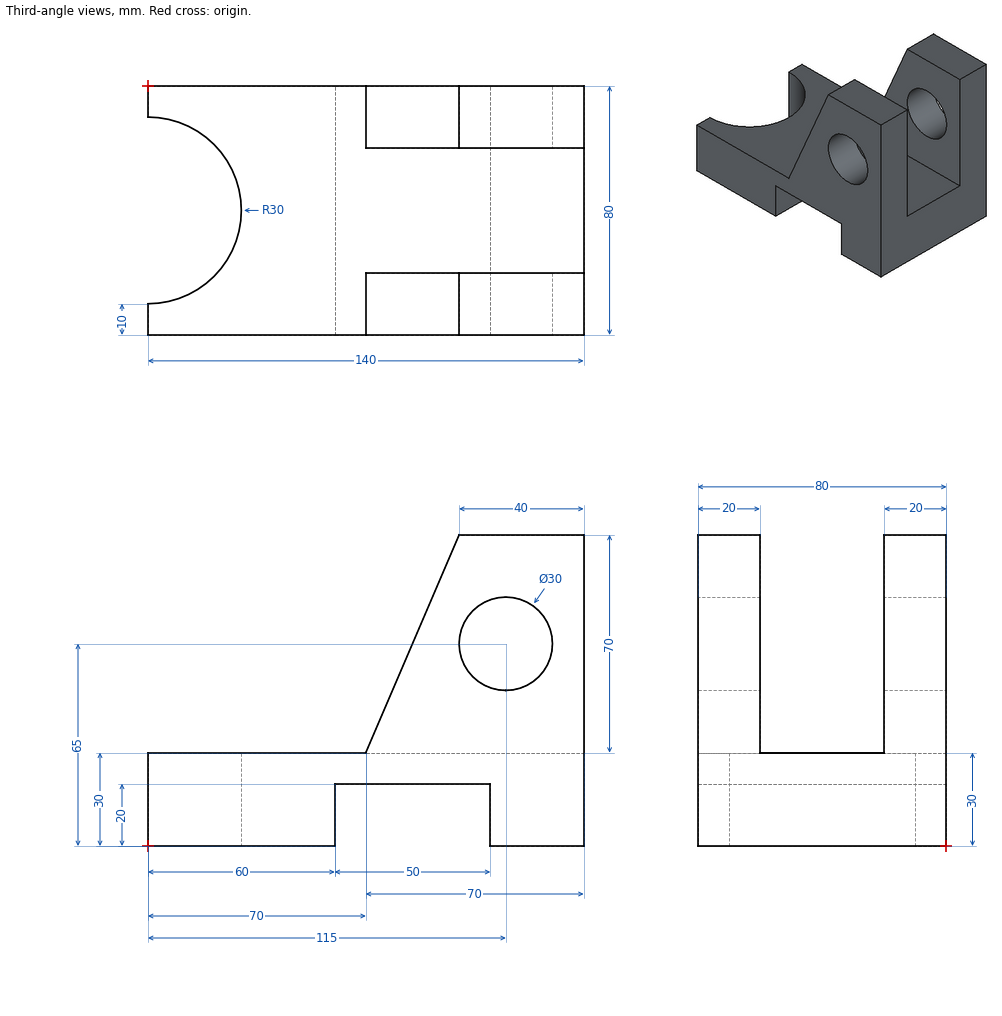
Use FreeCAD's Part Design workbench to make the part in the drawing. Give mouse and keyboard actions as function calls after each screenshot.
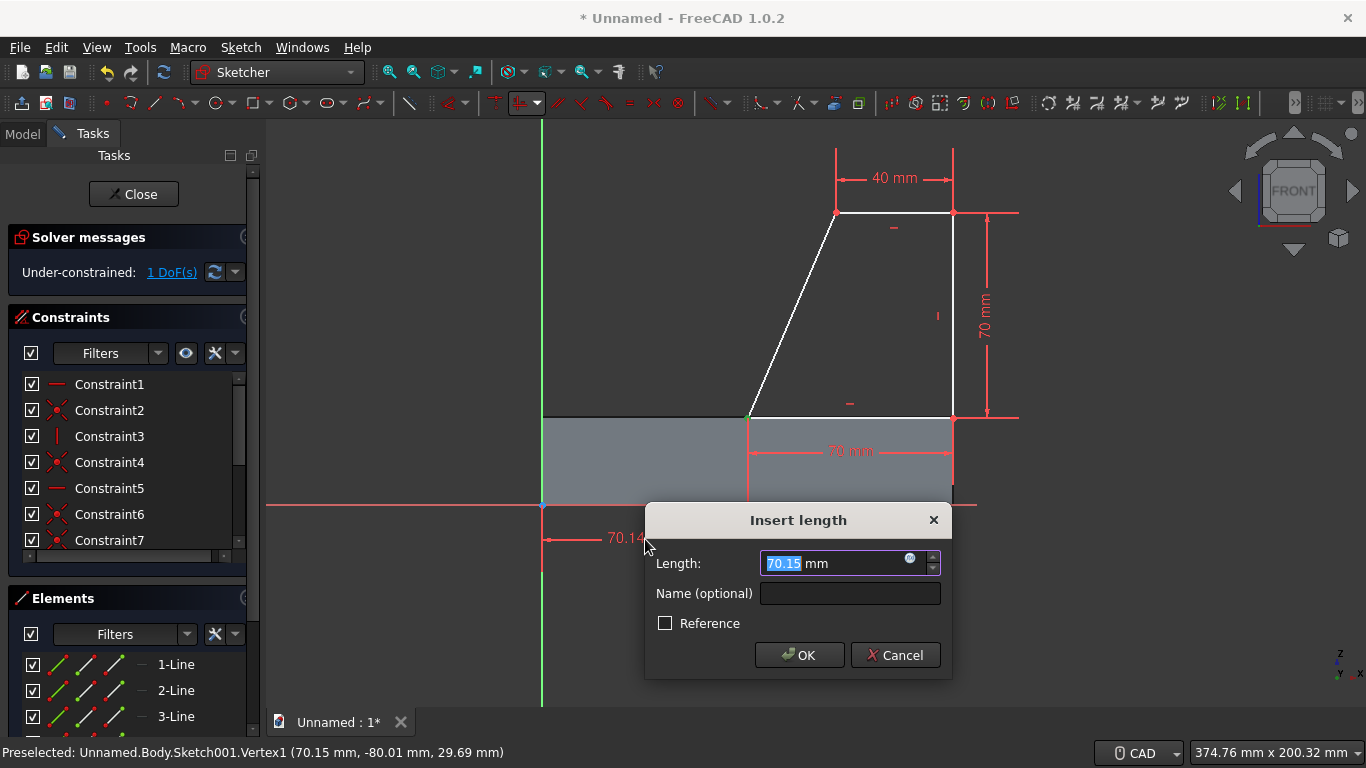
text(70)
key(Return)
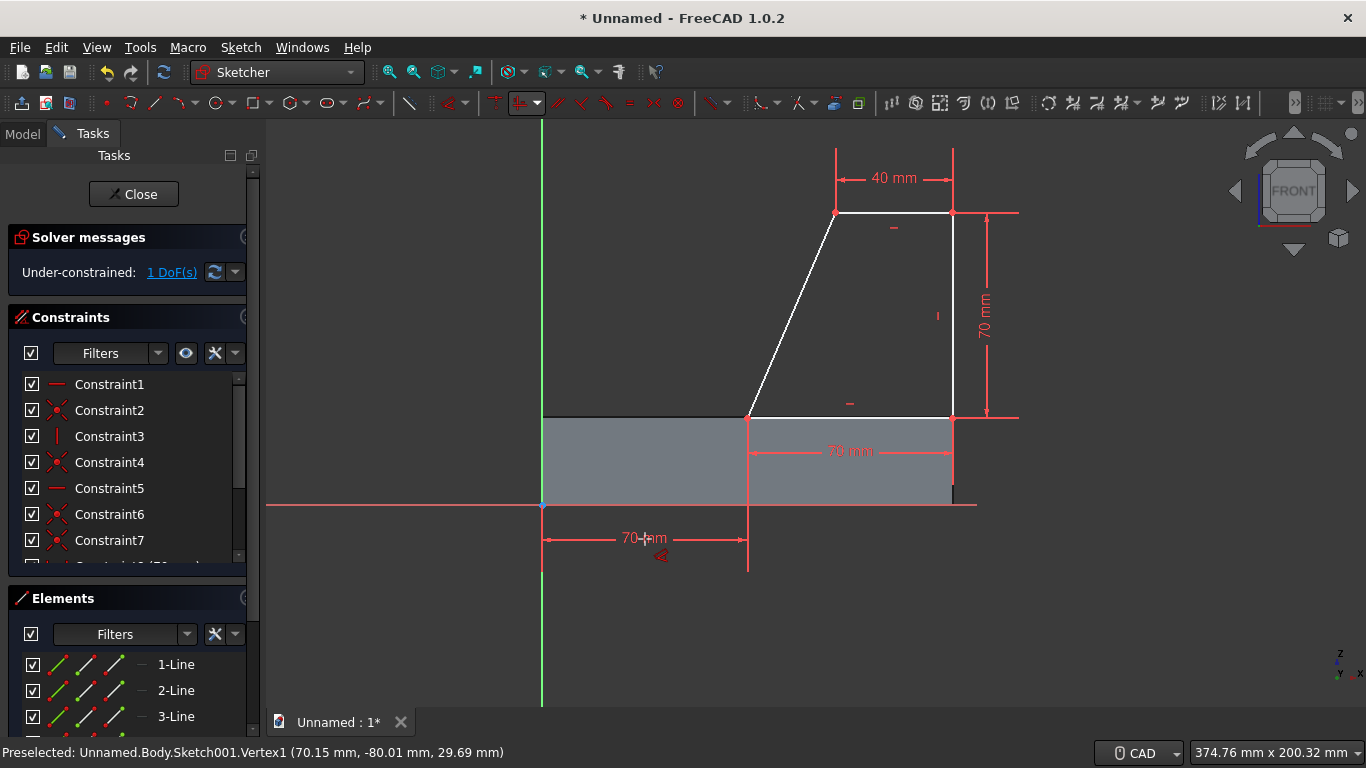
click(748, 418)
click(508, 462)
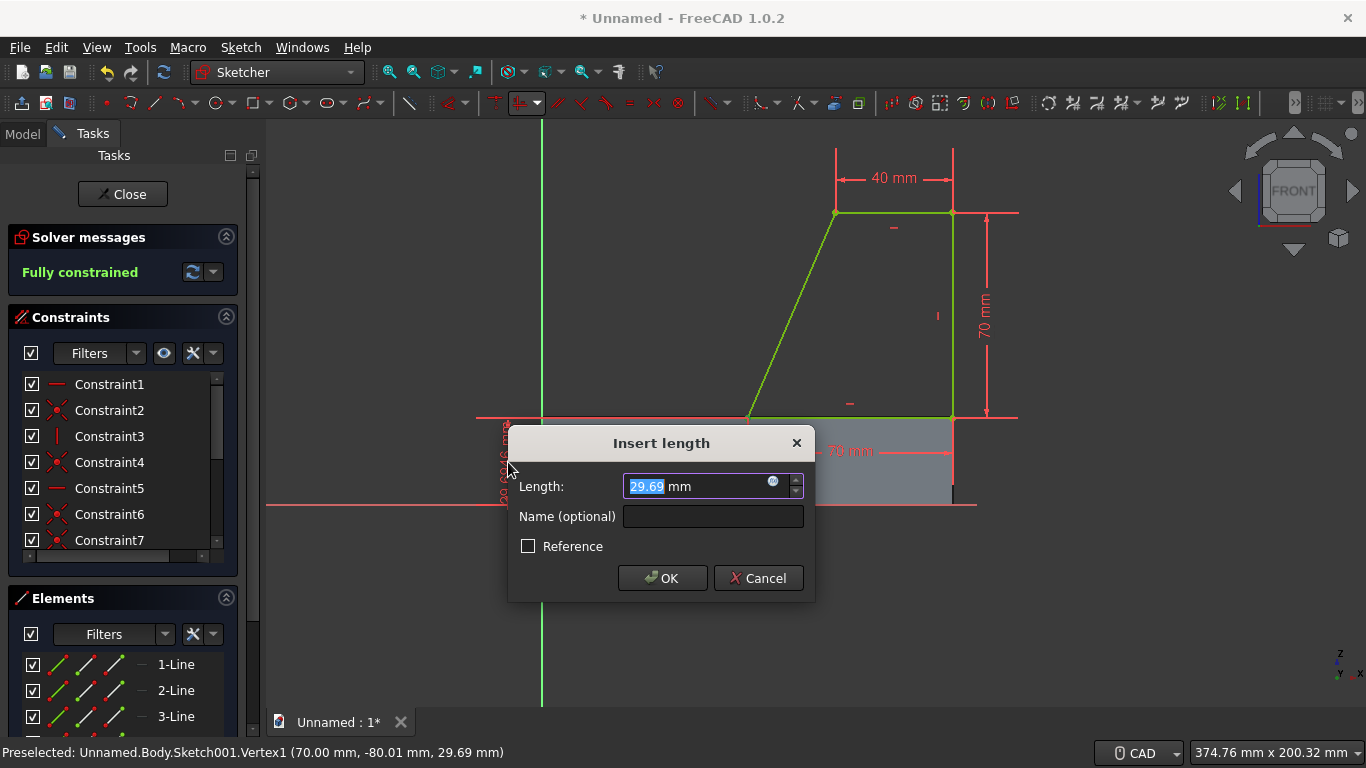
text(30)
key(Return)
key(Escape)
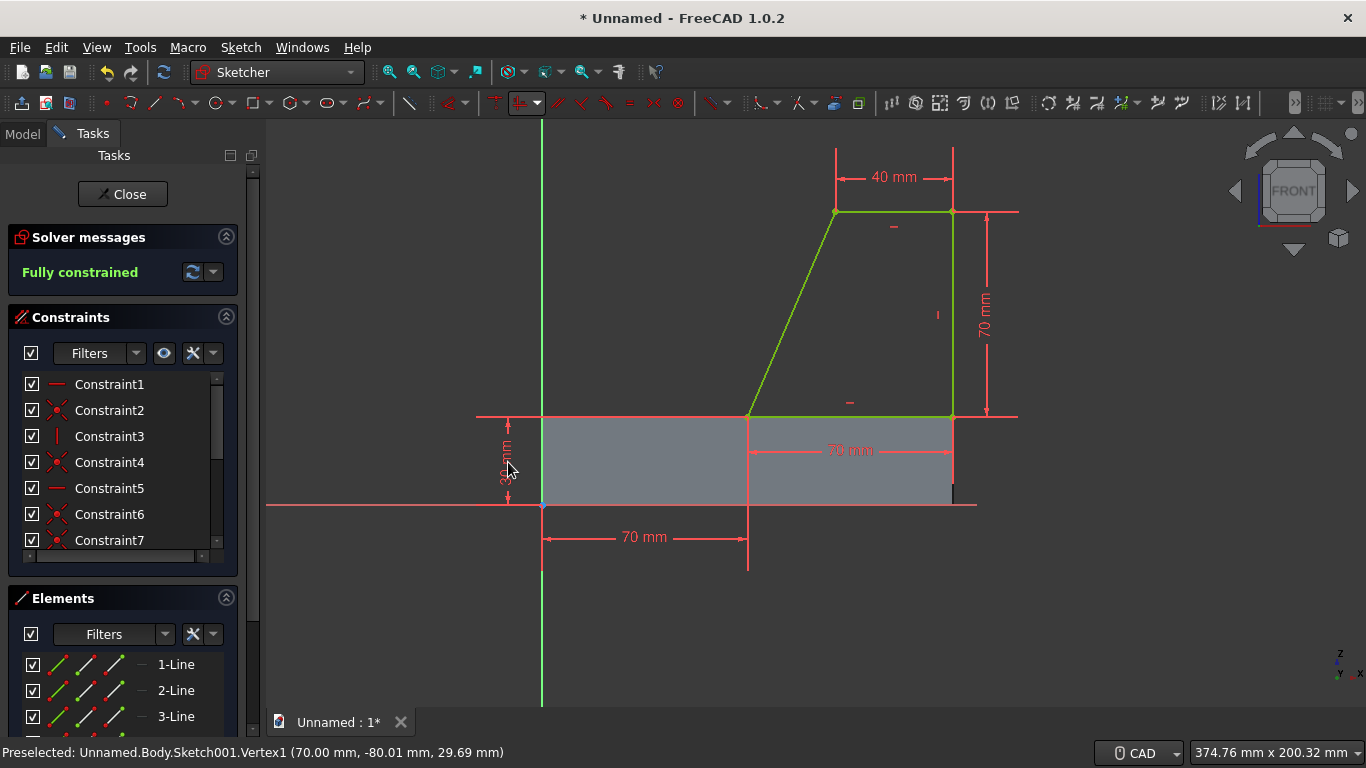
click(123, 194)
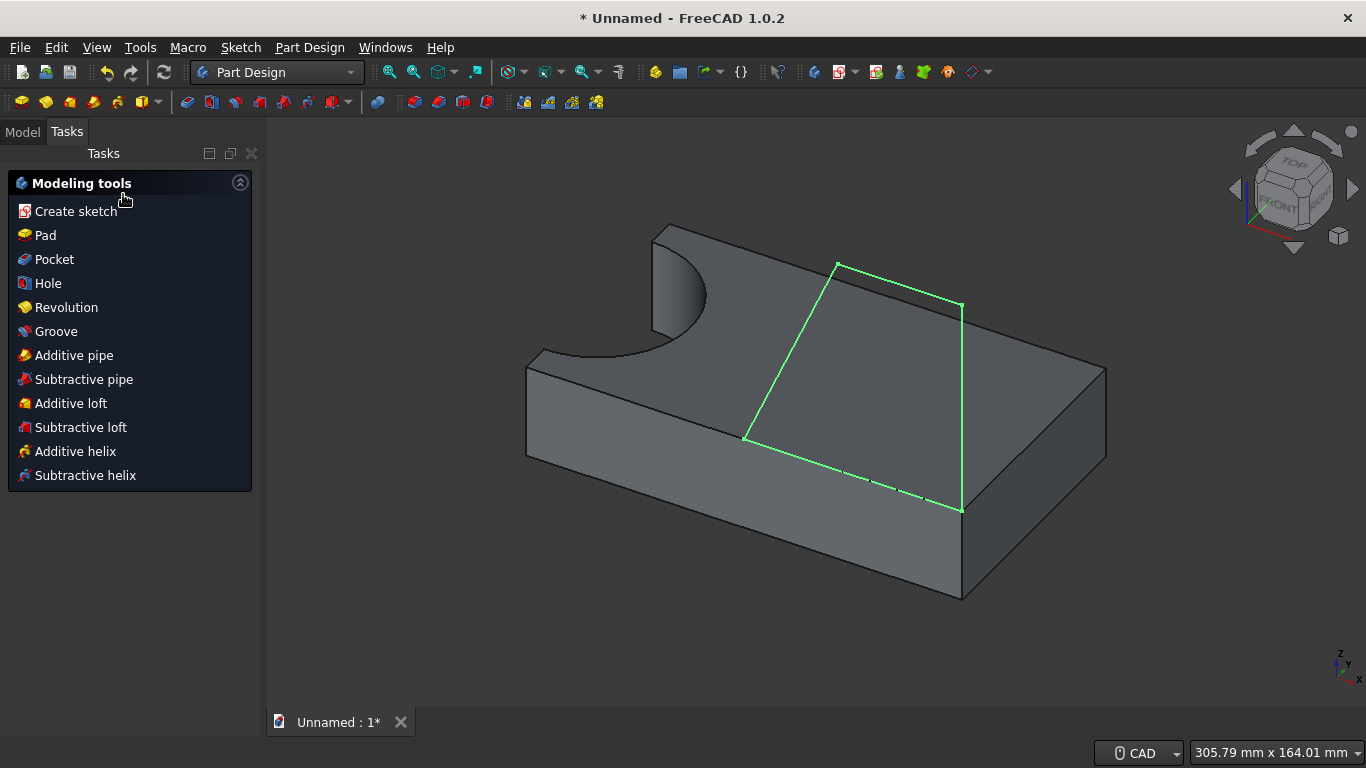
click(22, 102)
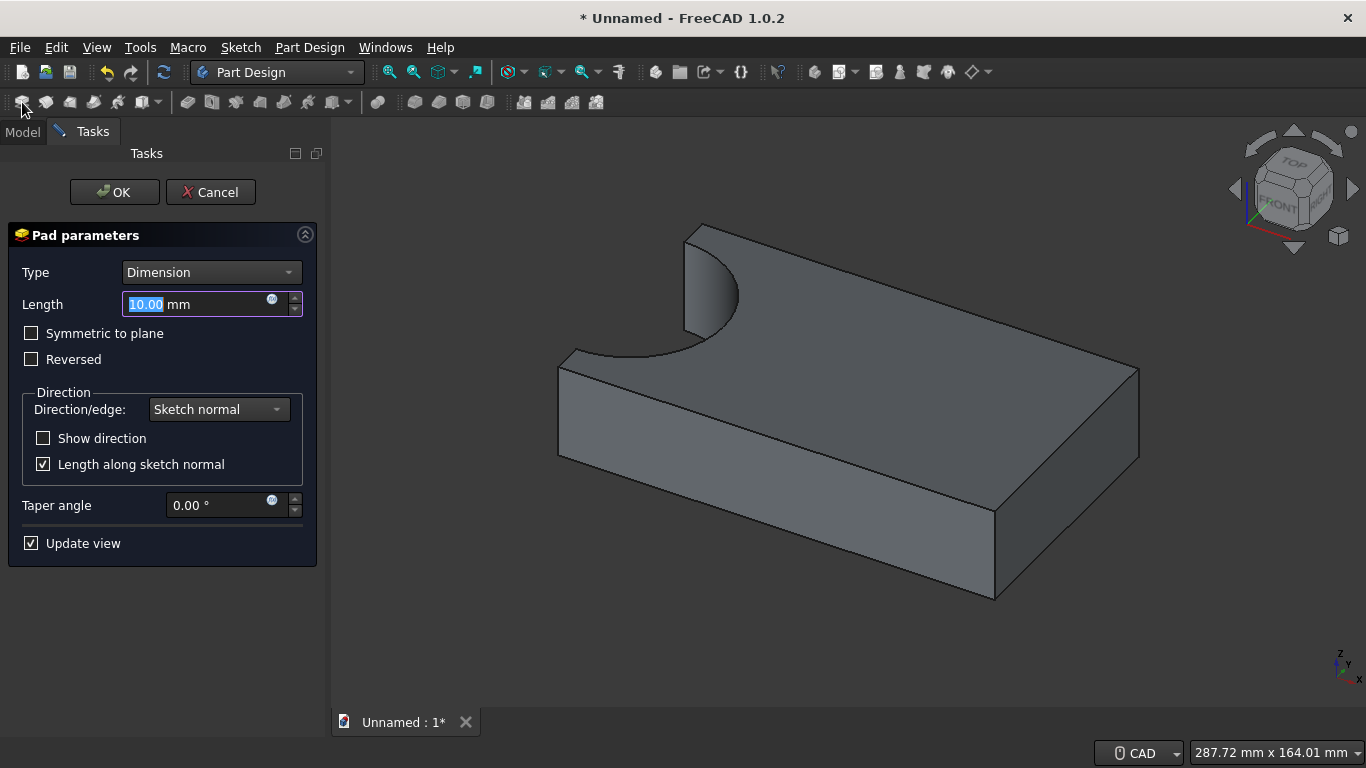
text(20)
key(Tab)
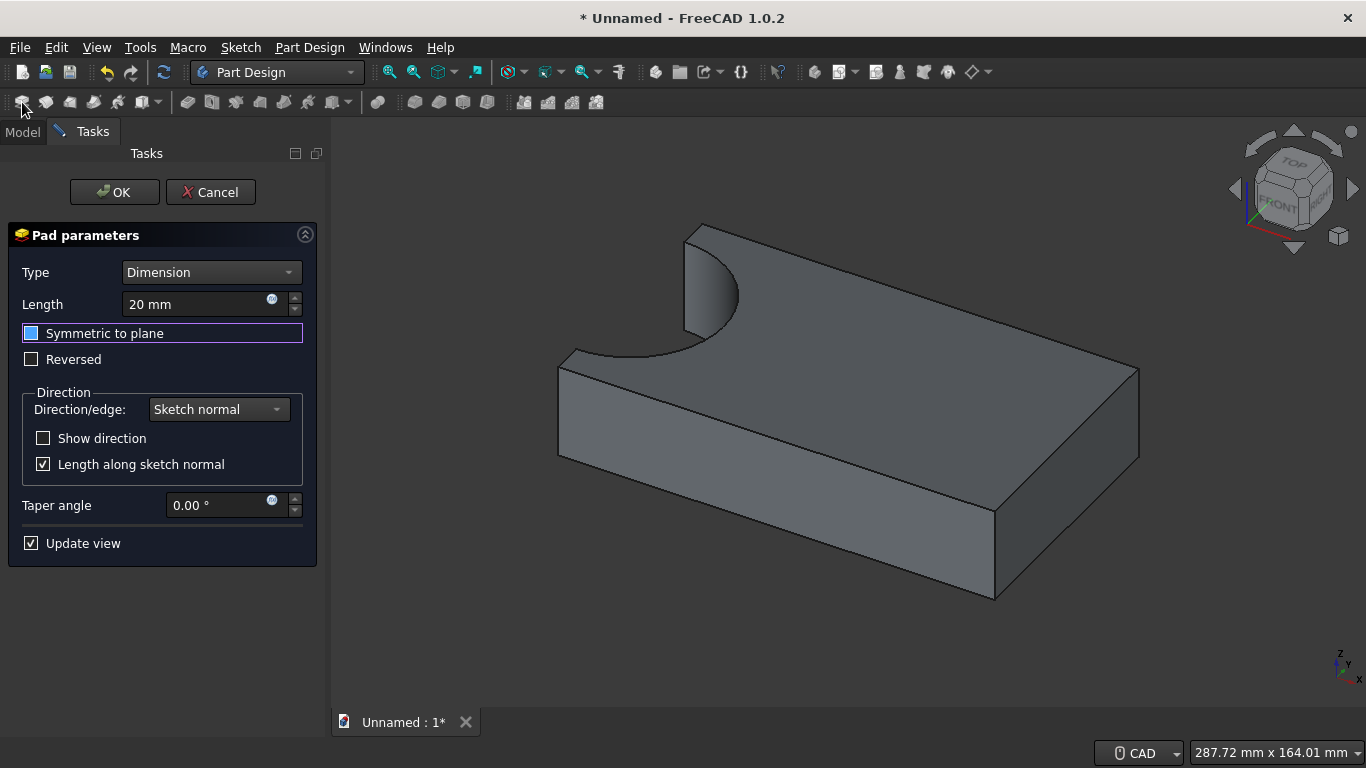
click(30, 359)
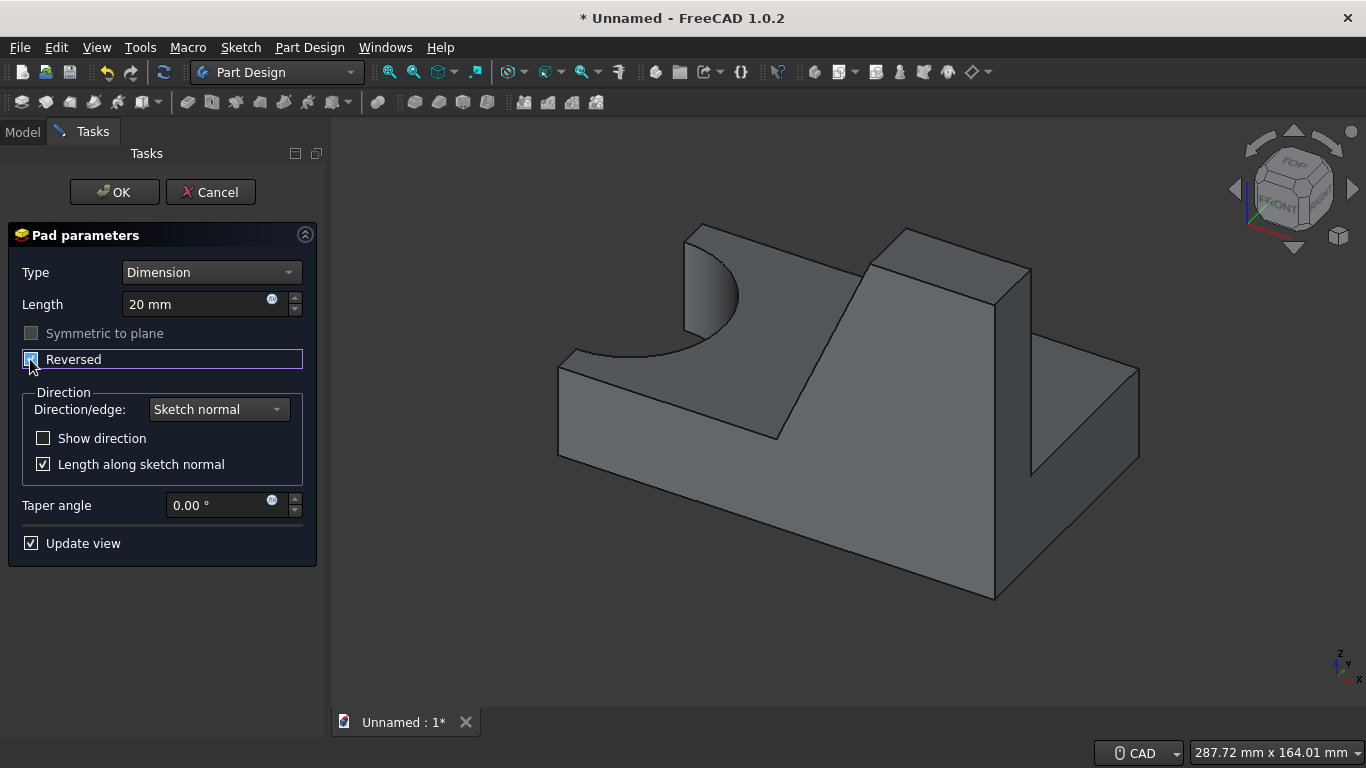
click(115, 192)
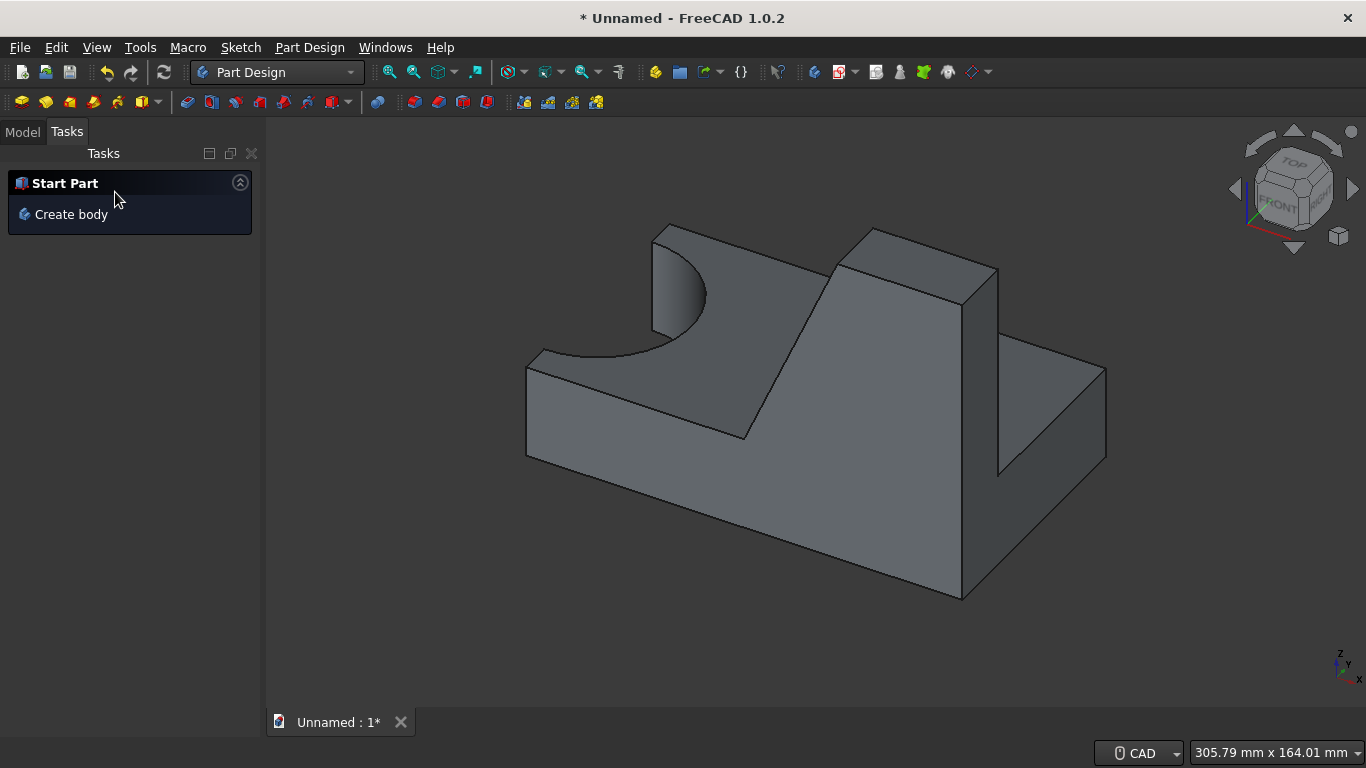
click(390, 72)